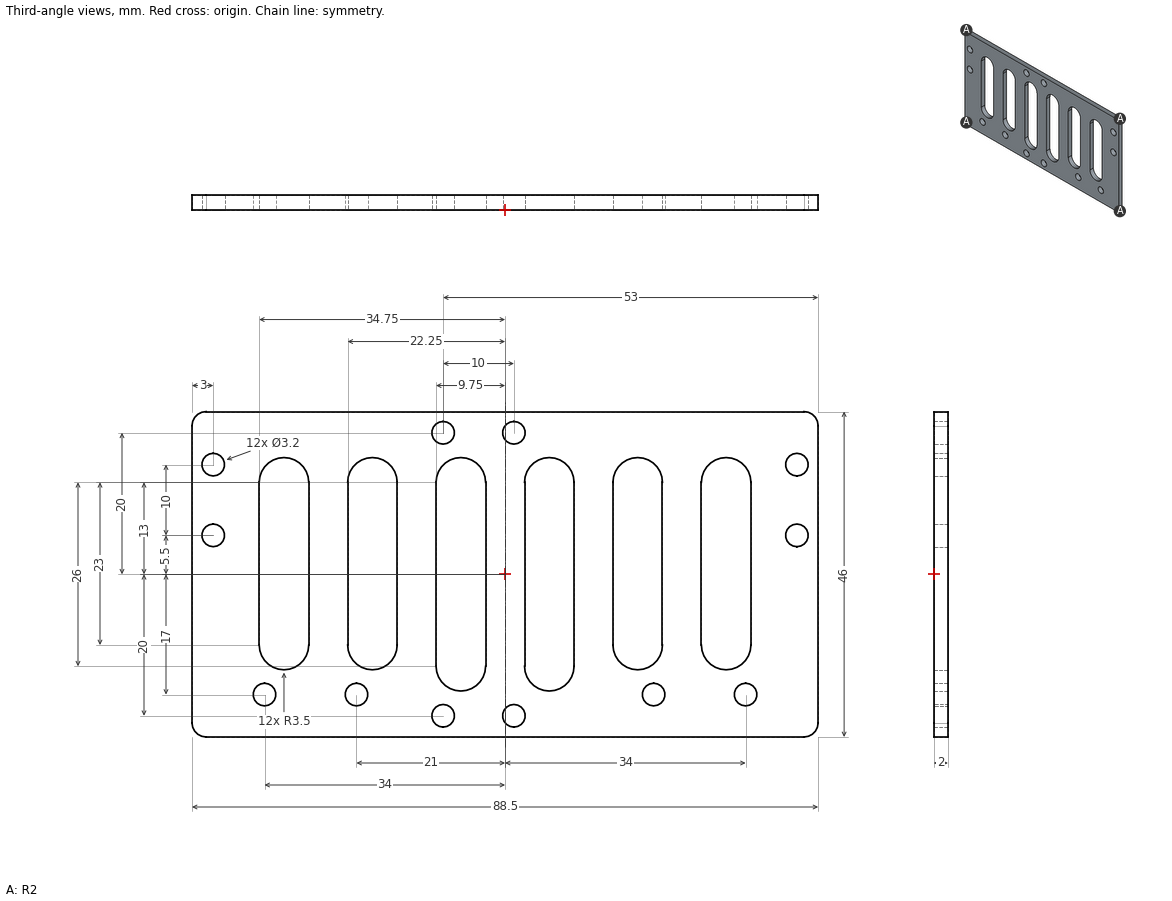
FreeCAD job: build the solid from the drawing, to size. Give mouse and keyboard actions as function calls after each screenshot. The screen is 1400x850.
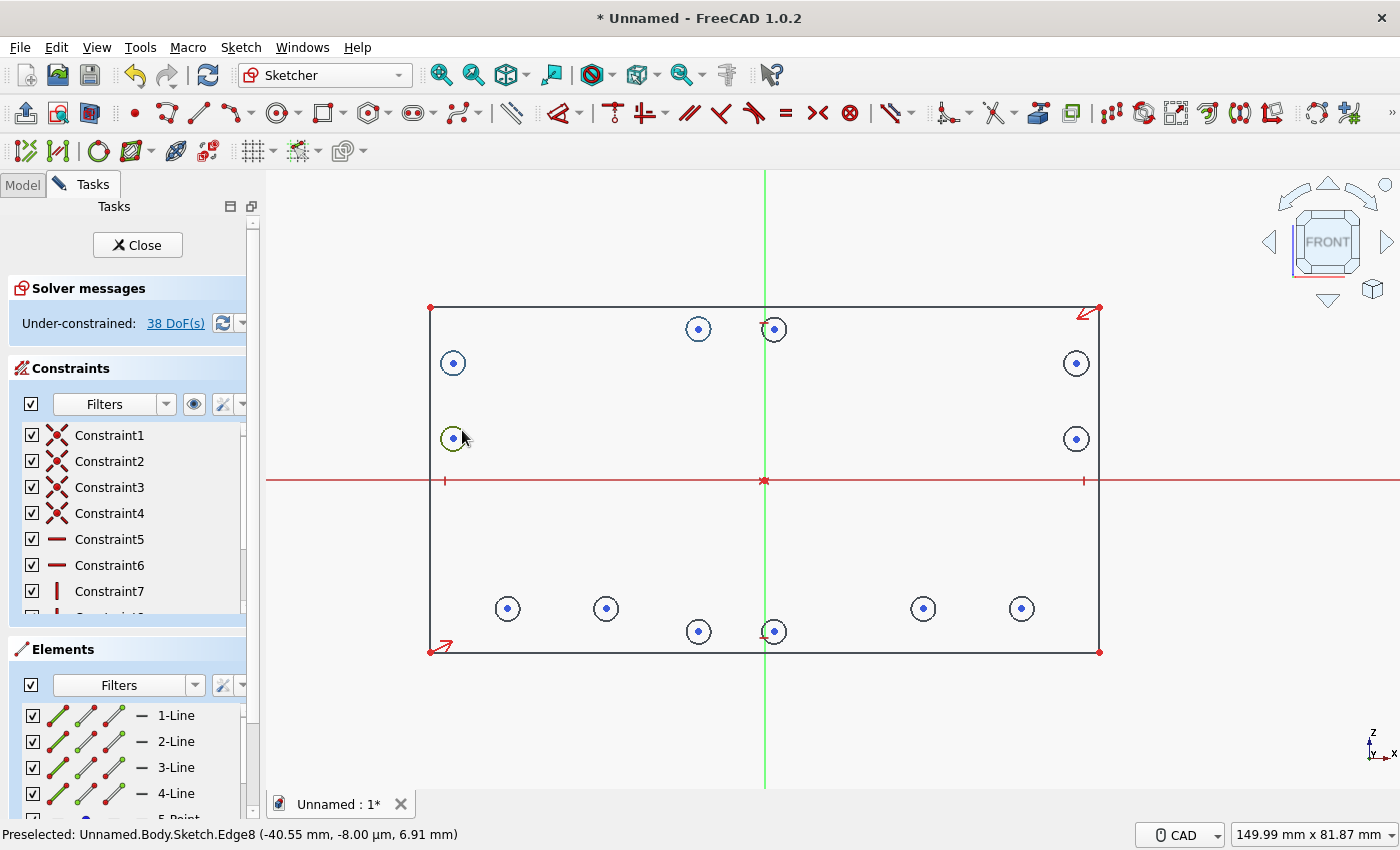
click(783, 321)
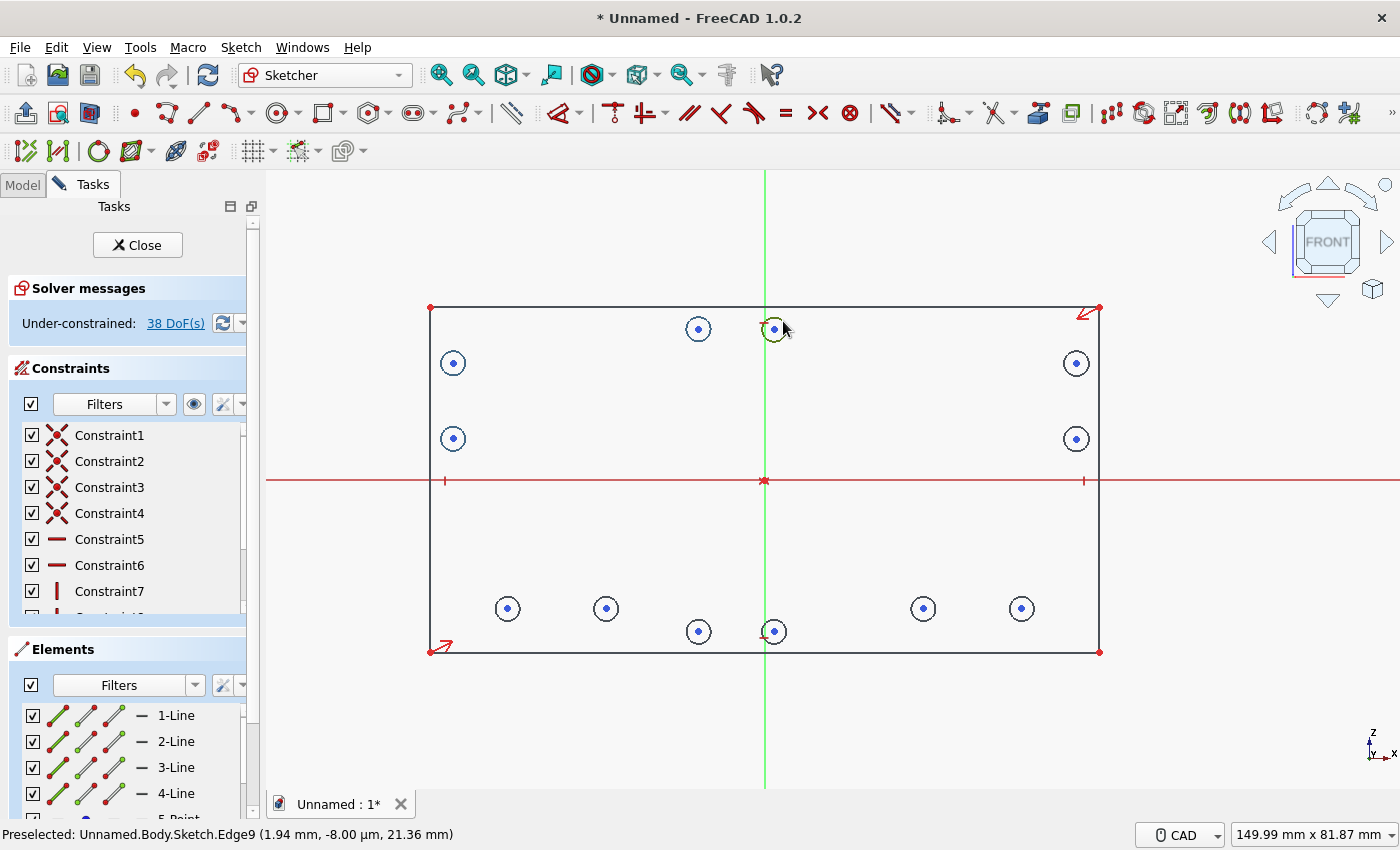
click(1085, 355)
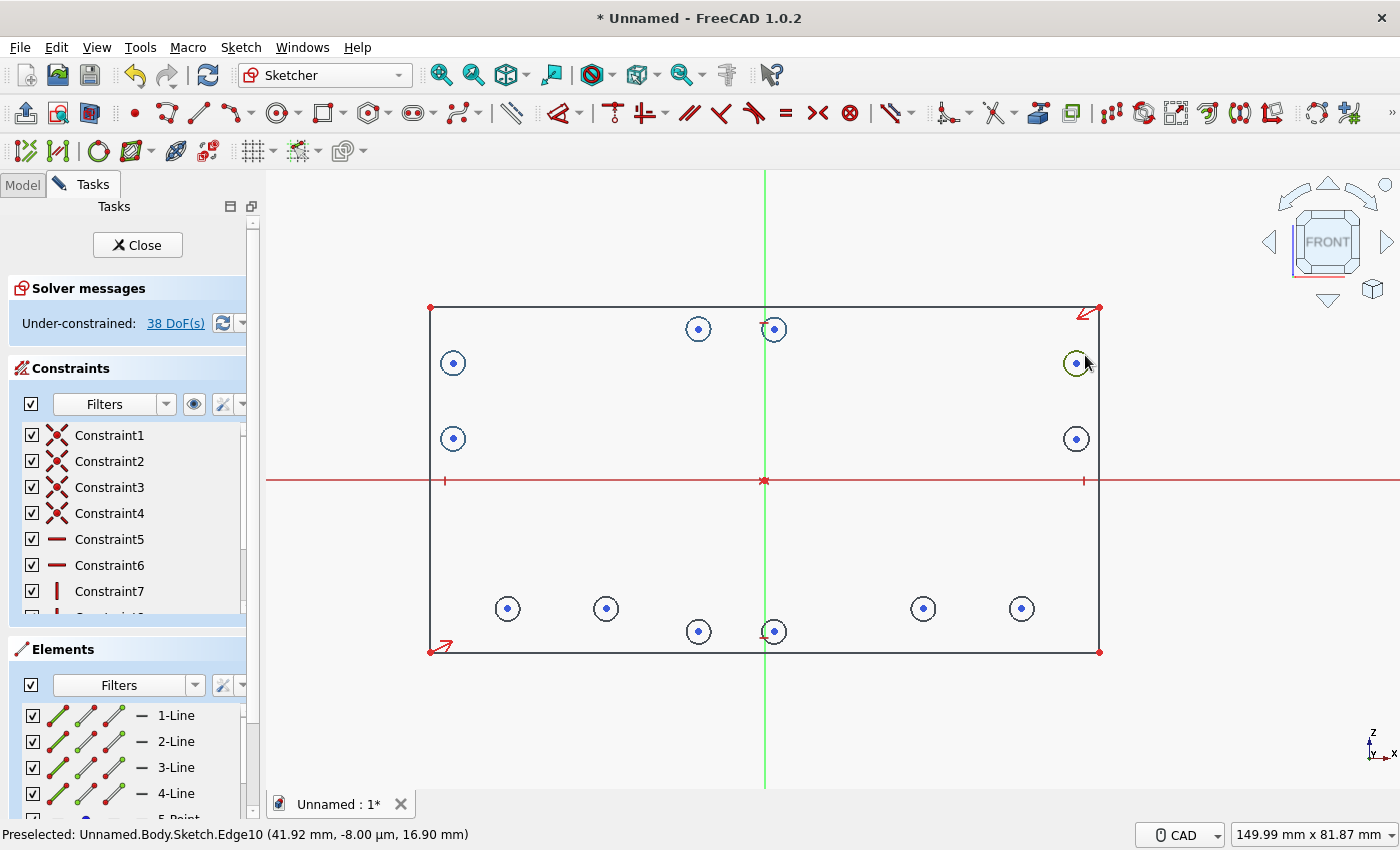
click(1085, 430)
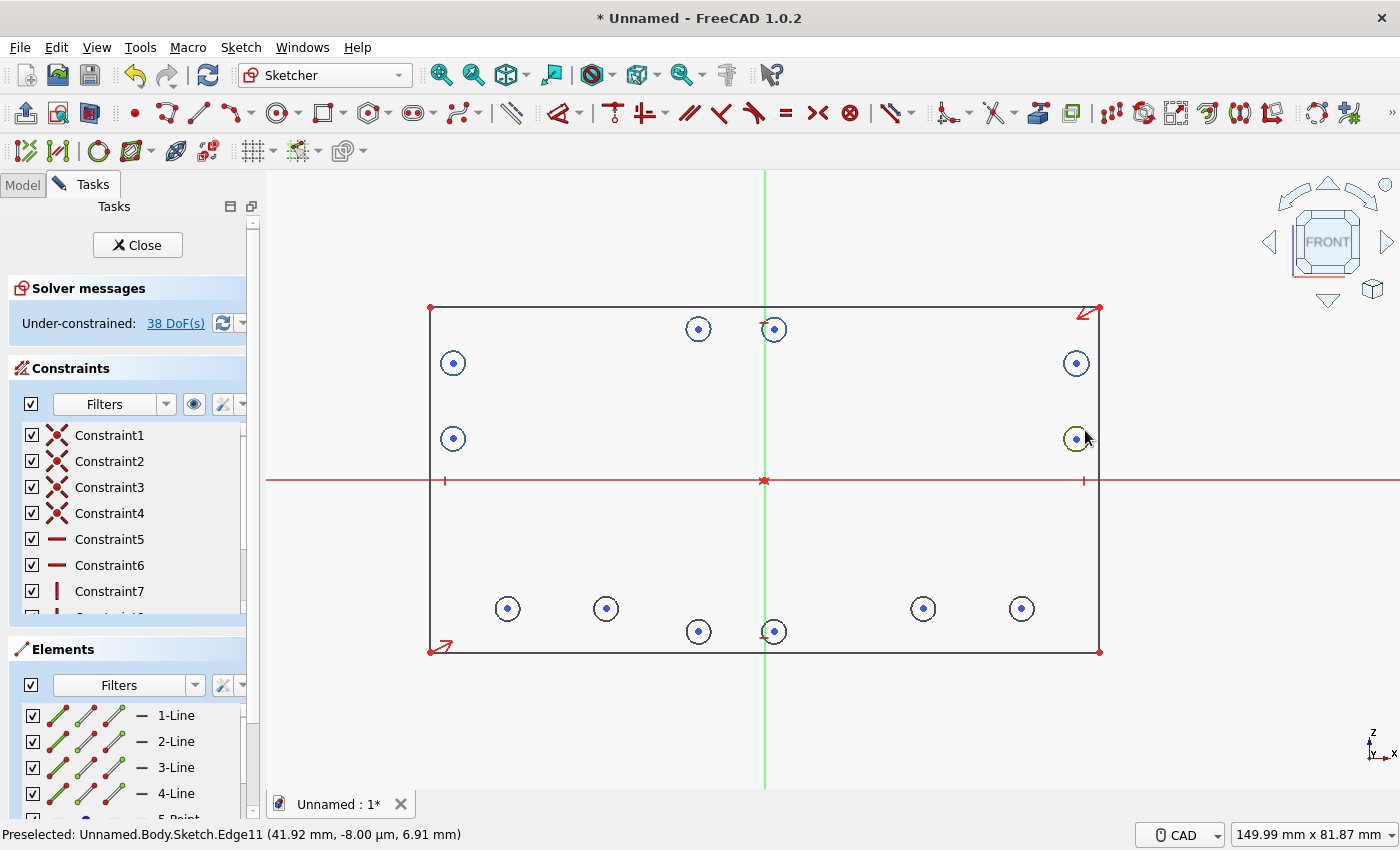
click(516, 600)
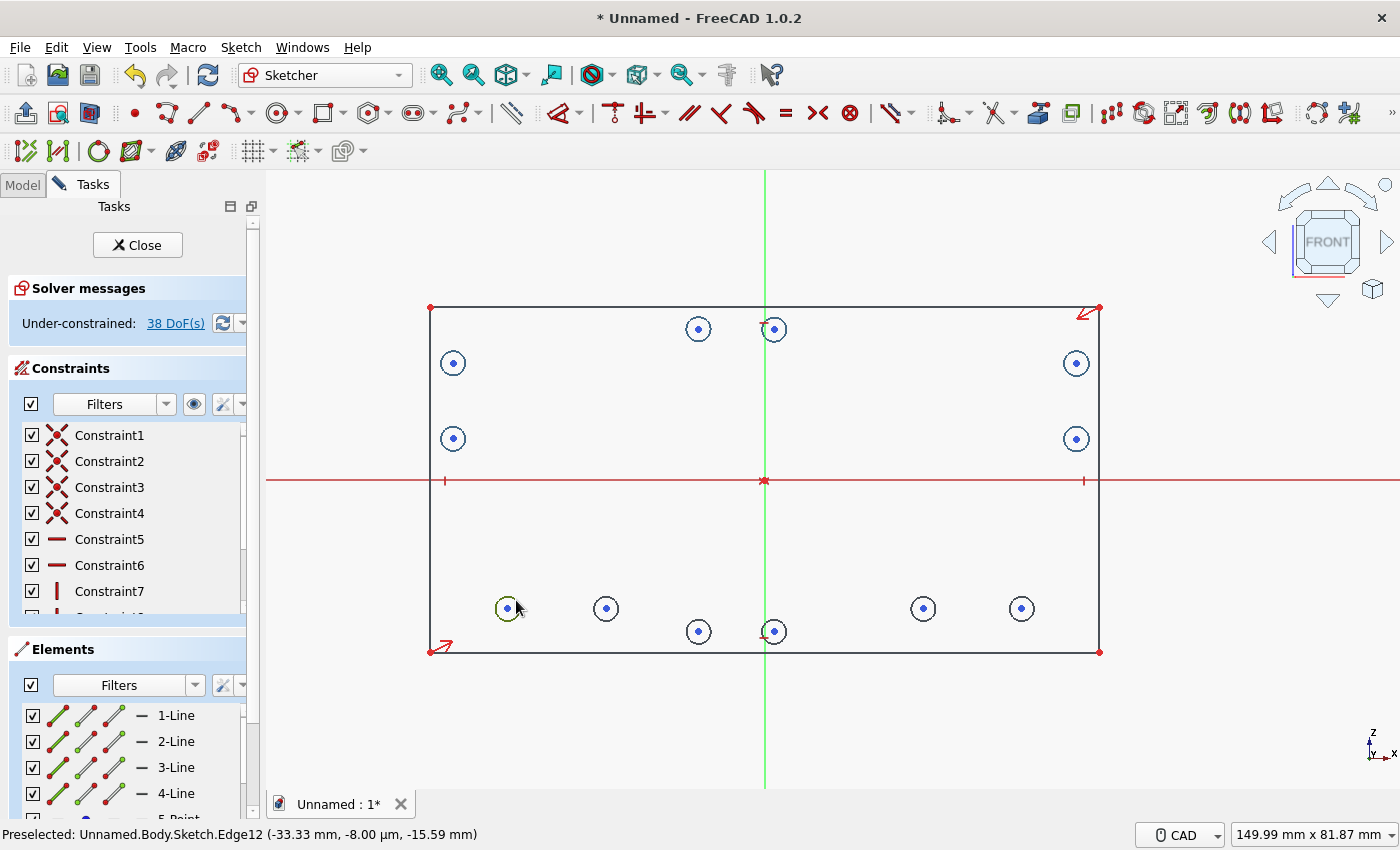
click(615, 600)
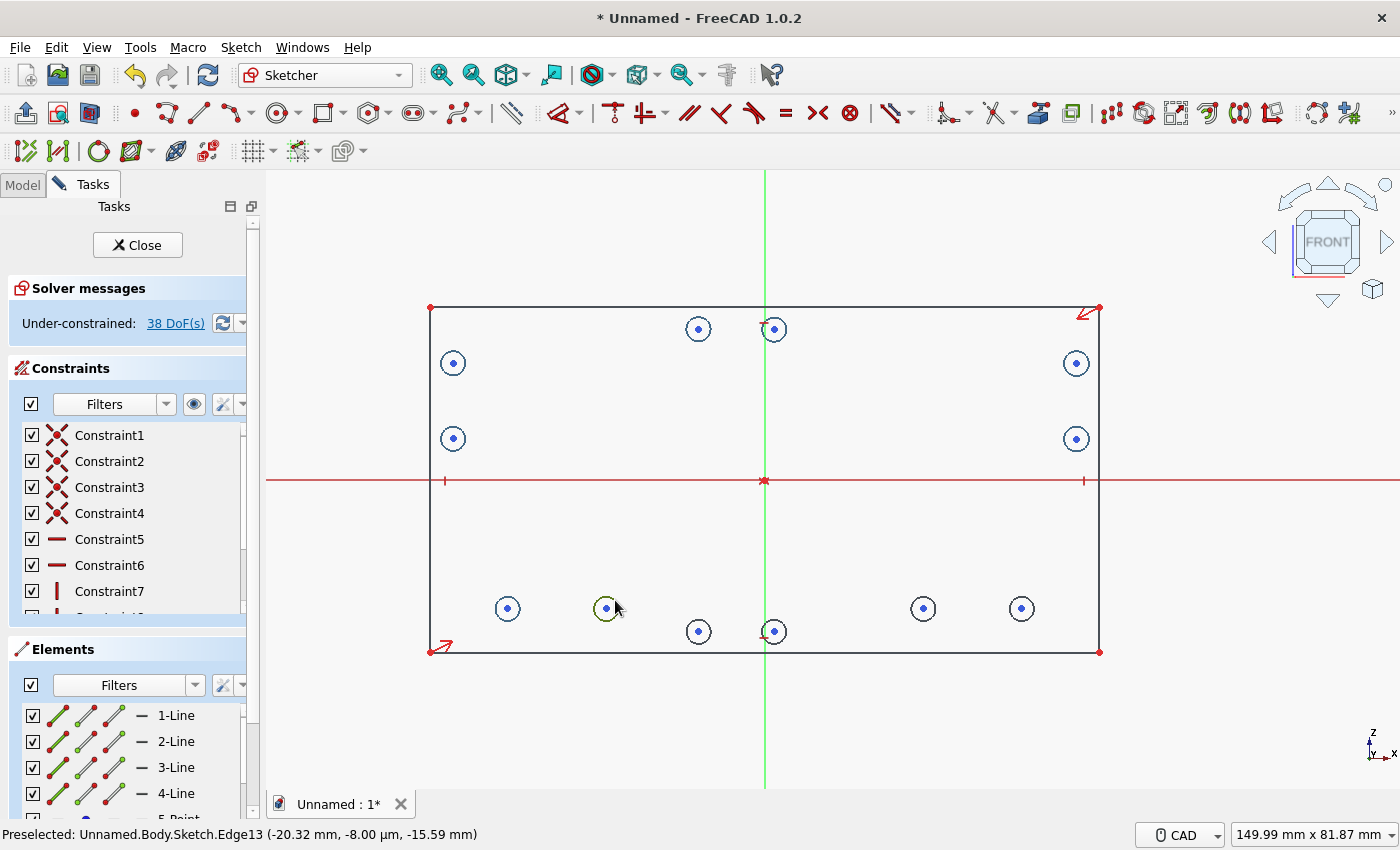
click(707, 623)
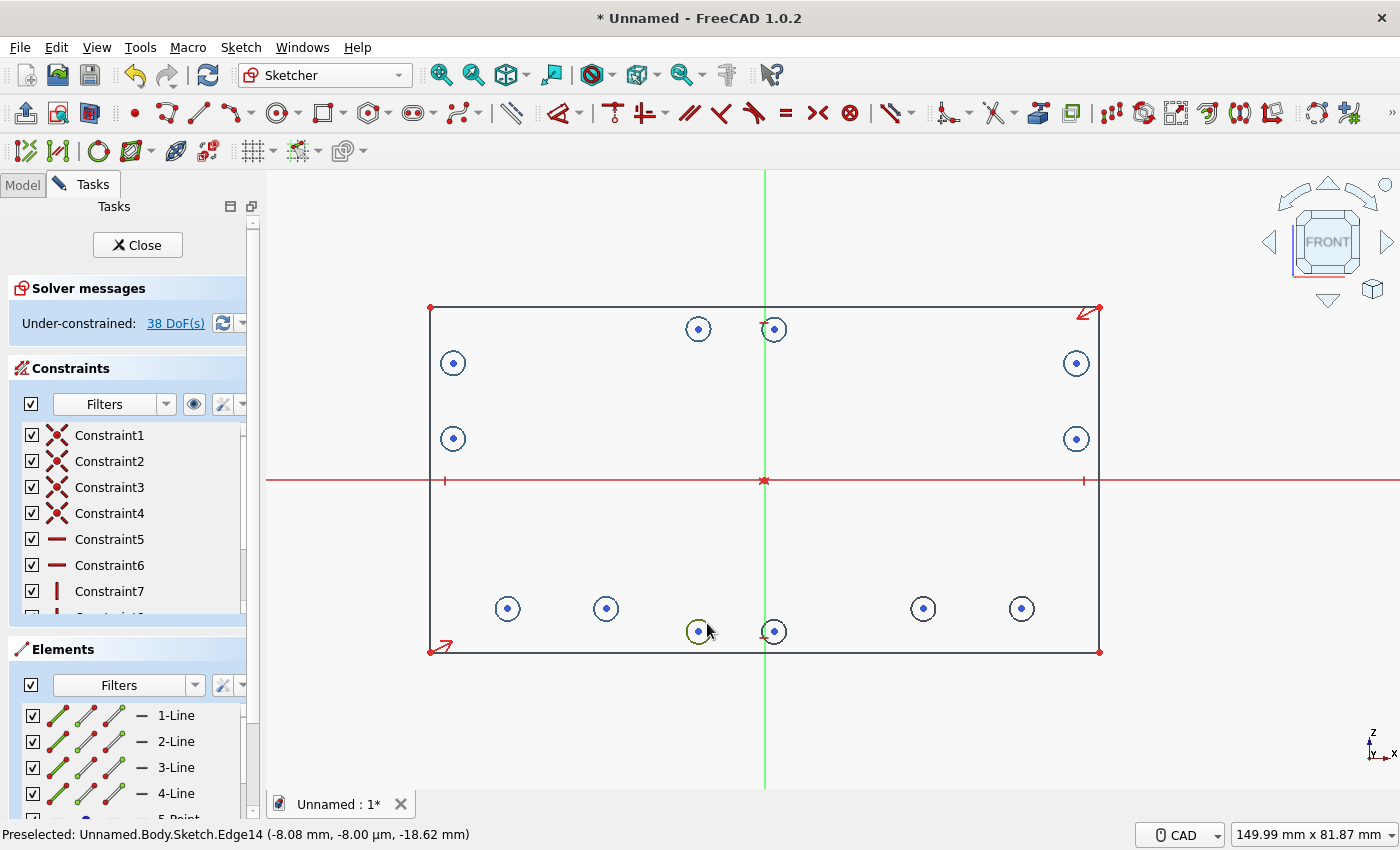
click(783, 623)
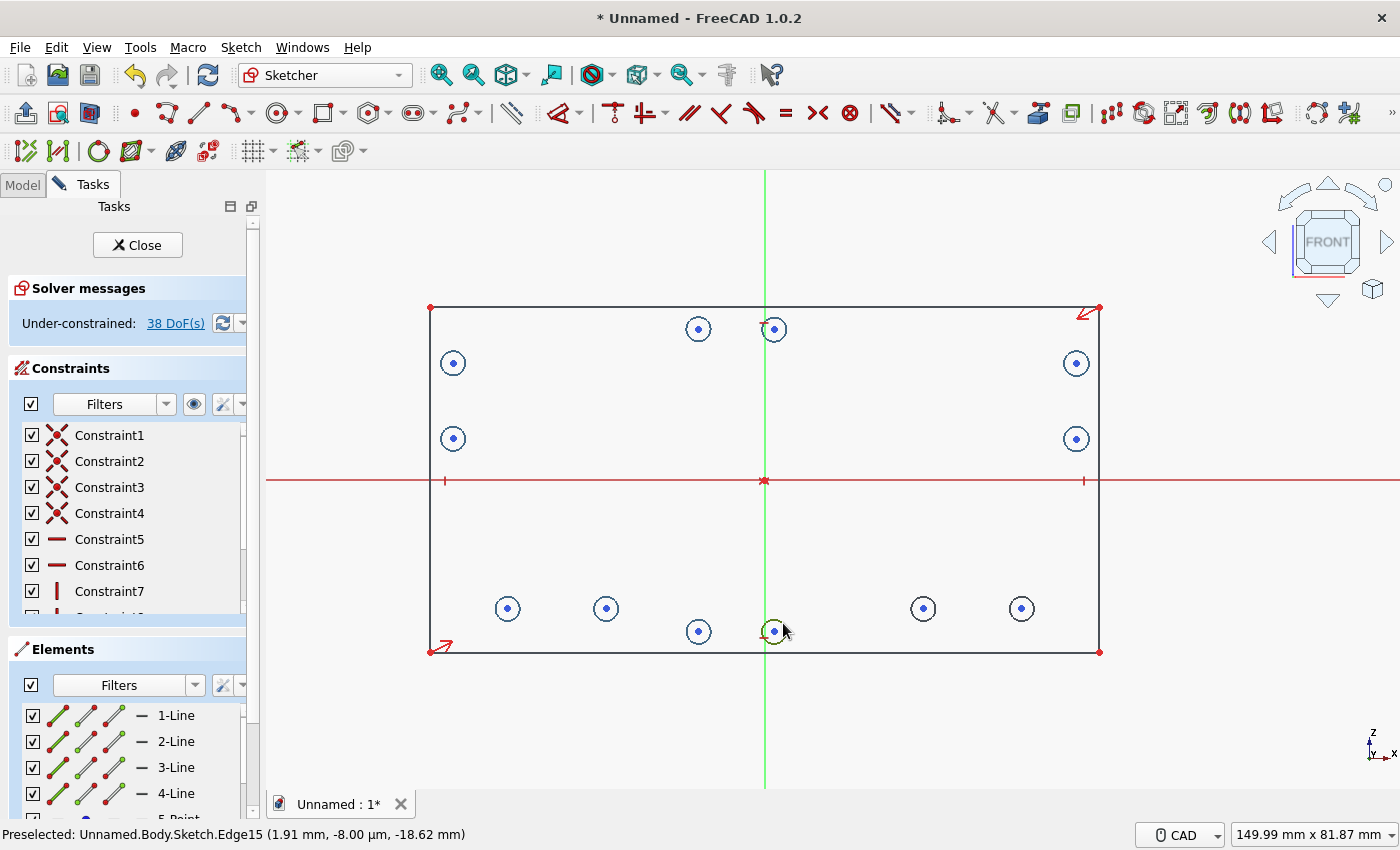
click(932, 600)